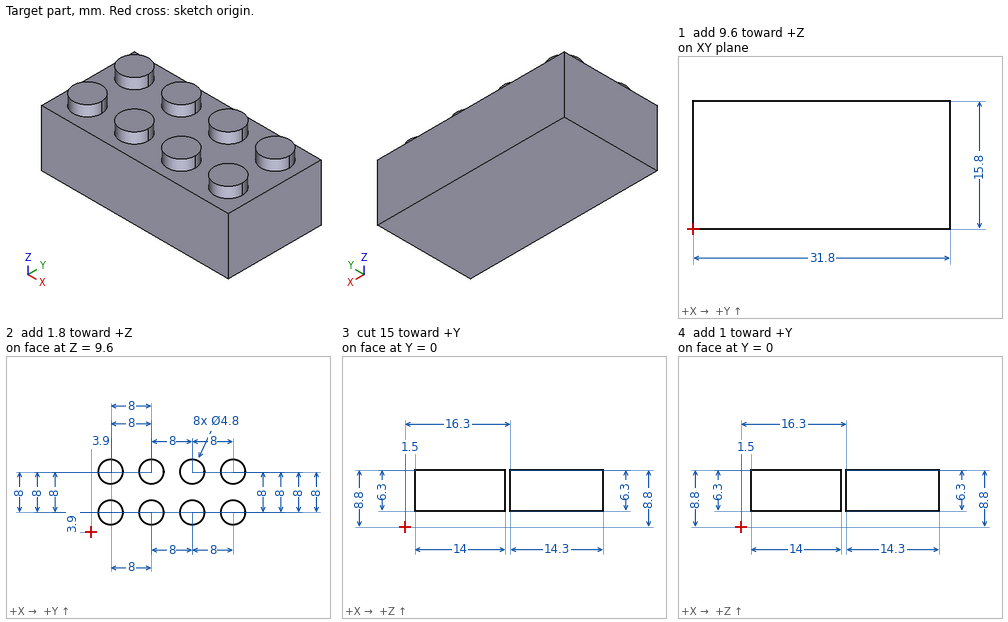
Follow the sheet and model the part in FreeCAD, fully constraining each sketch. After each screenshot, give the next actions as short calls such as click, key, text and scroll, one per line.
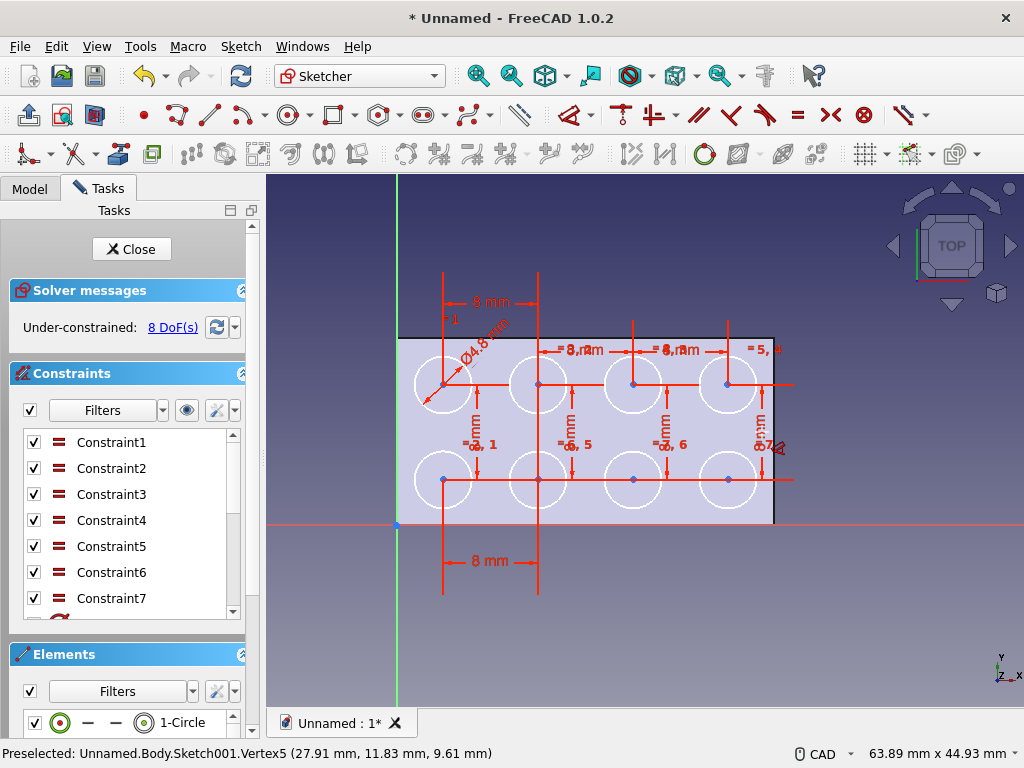
click(443, 480)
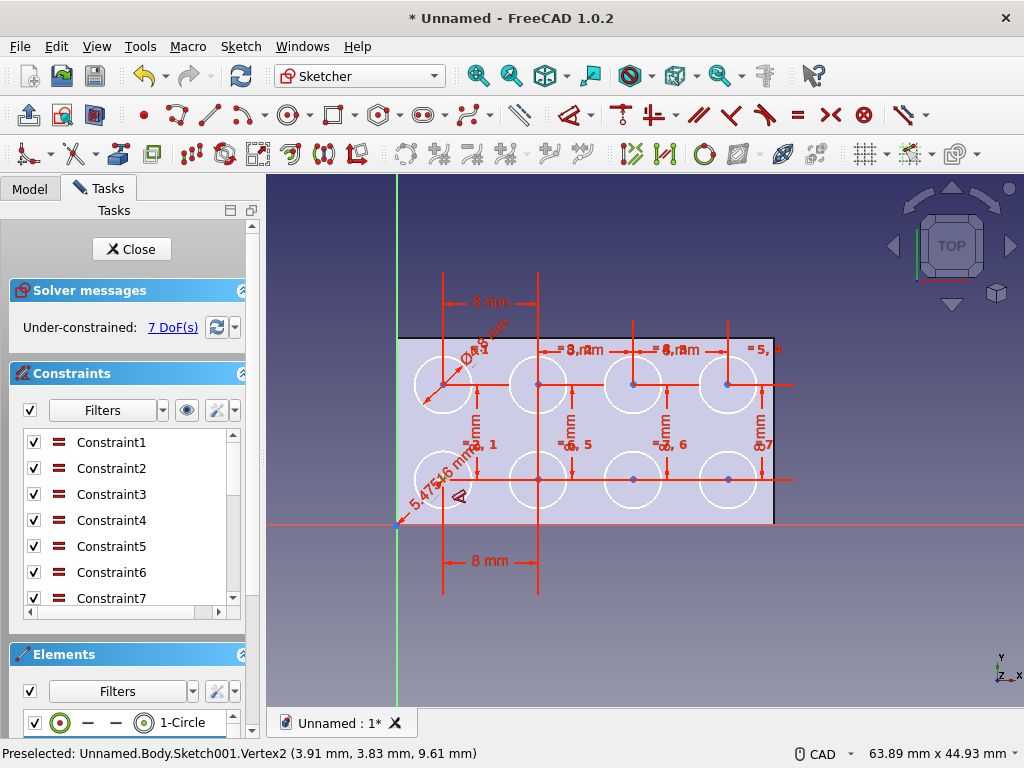
click(538, 480)
click(491, 398)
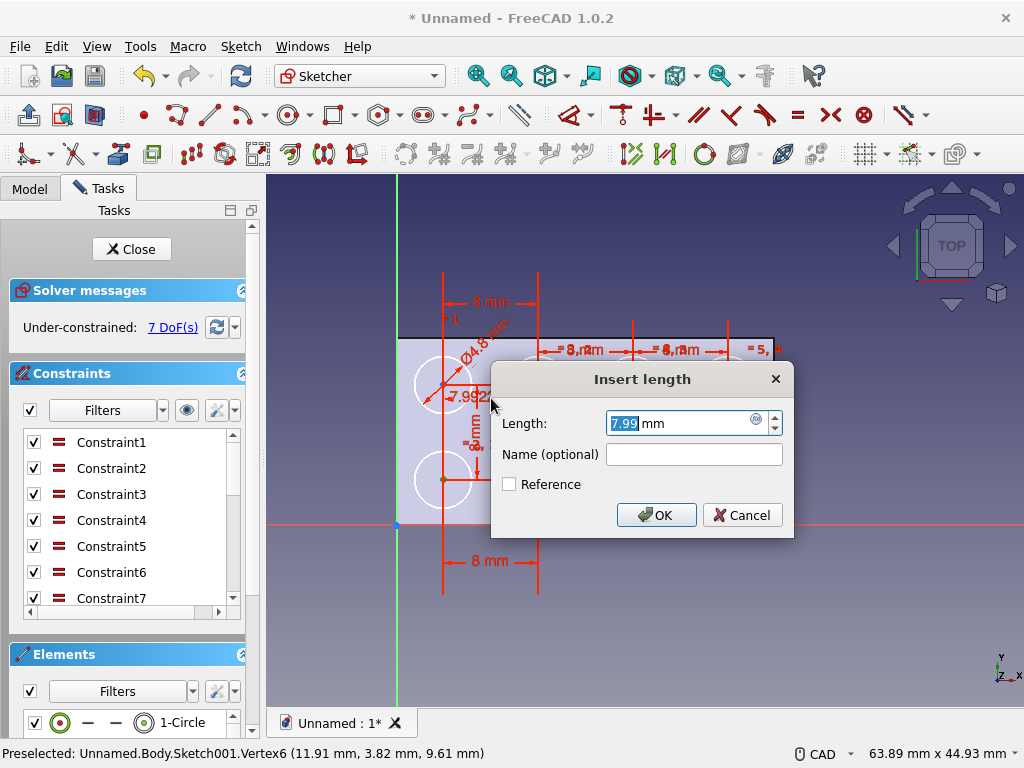
text(8)
key(Return)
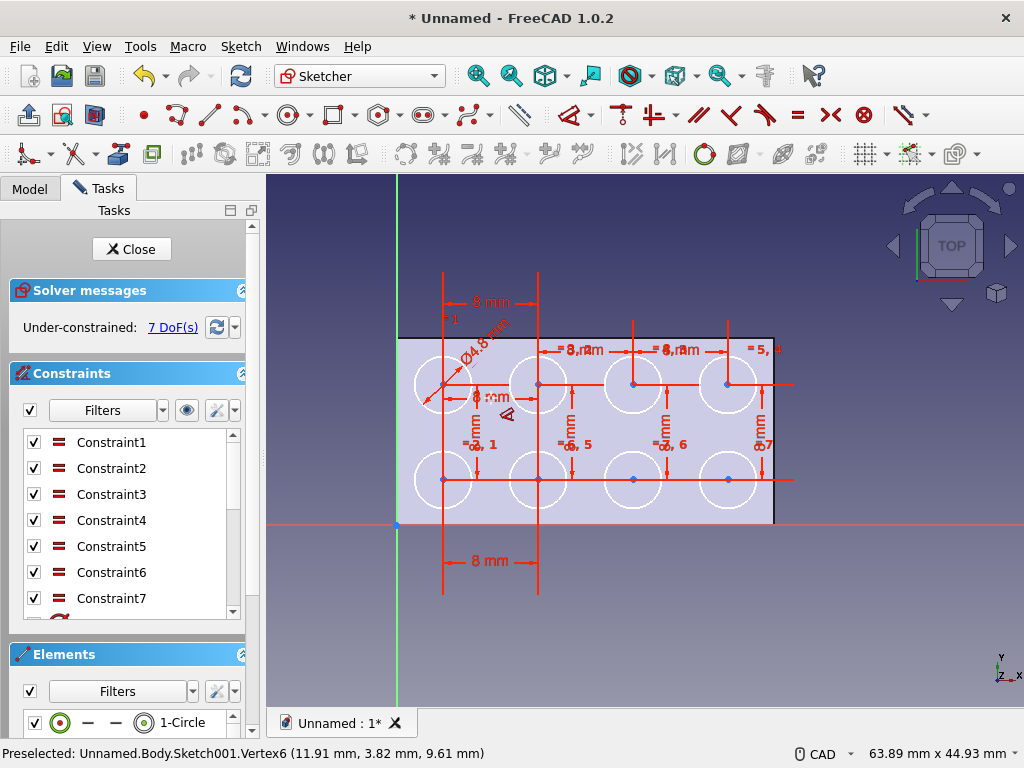
click(538, 385)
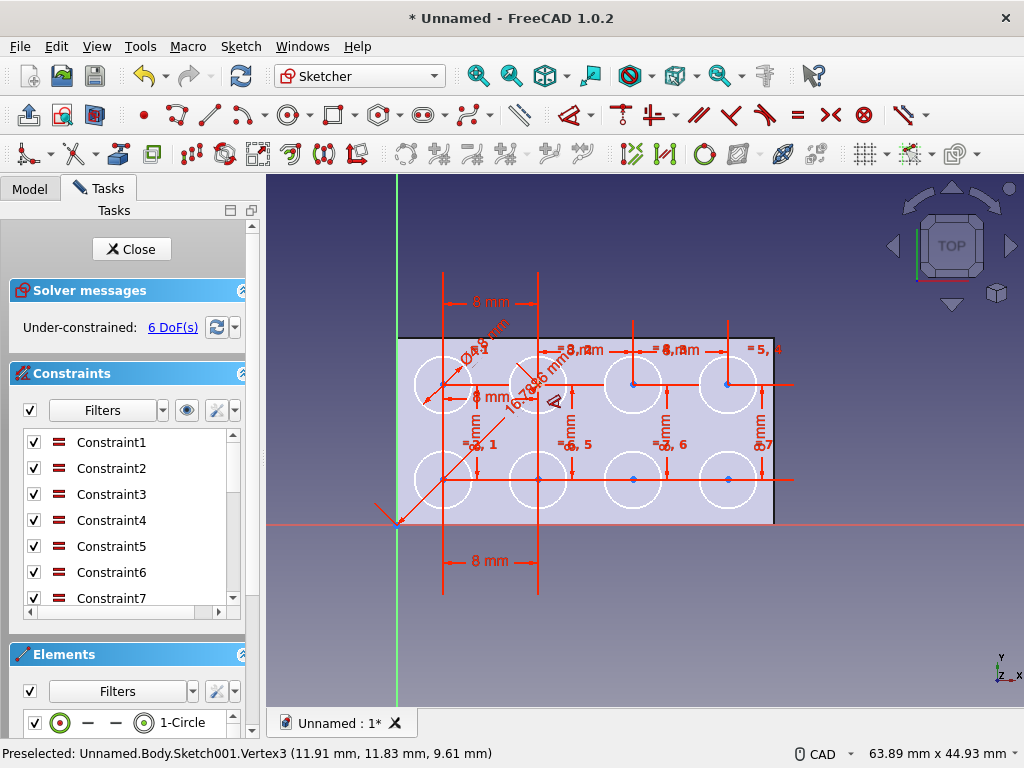
click(538, 480)
click(504, 454)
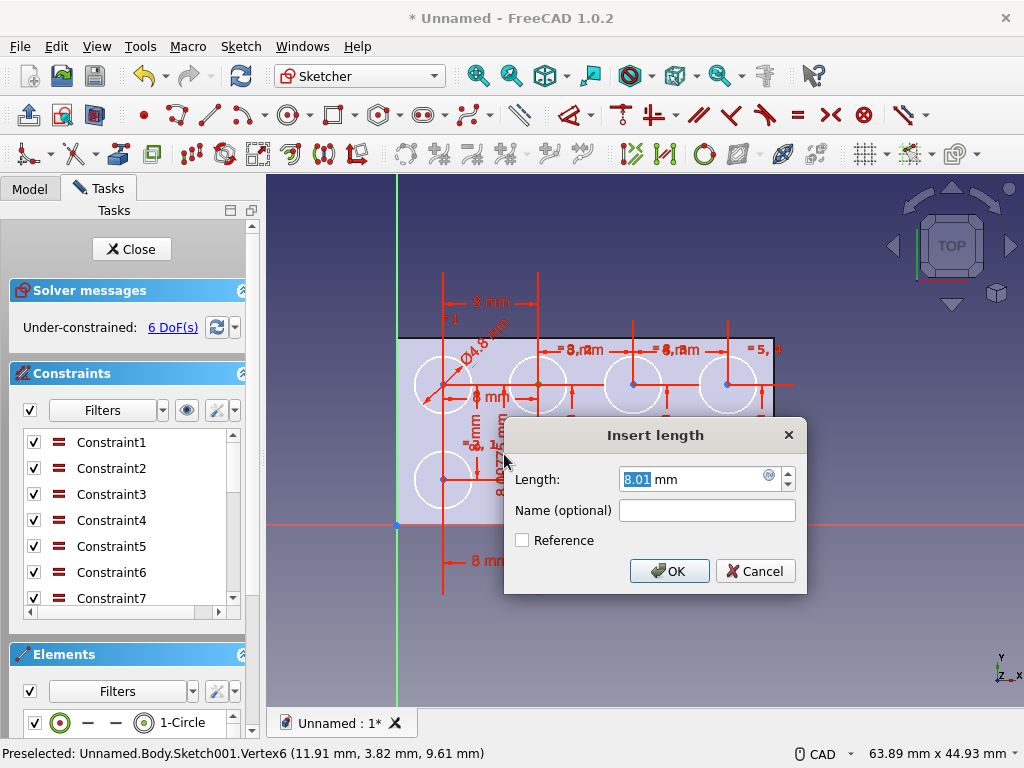
text(8)
key(Return)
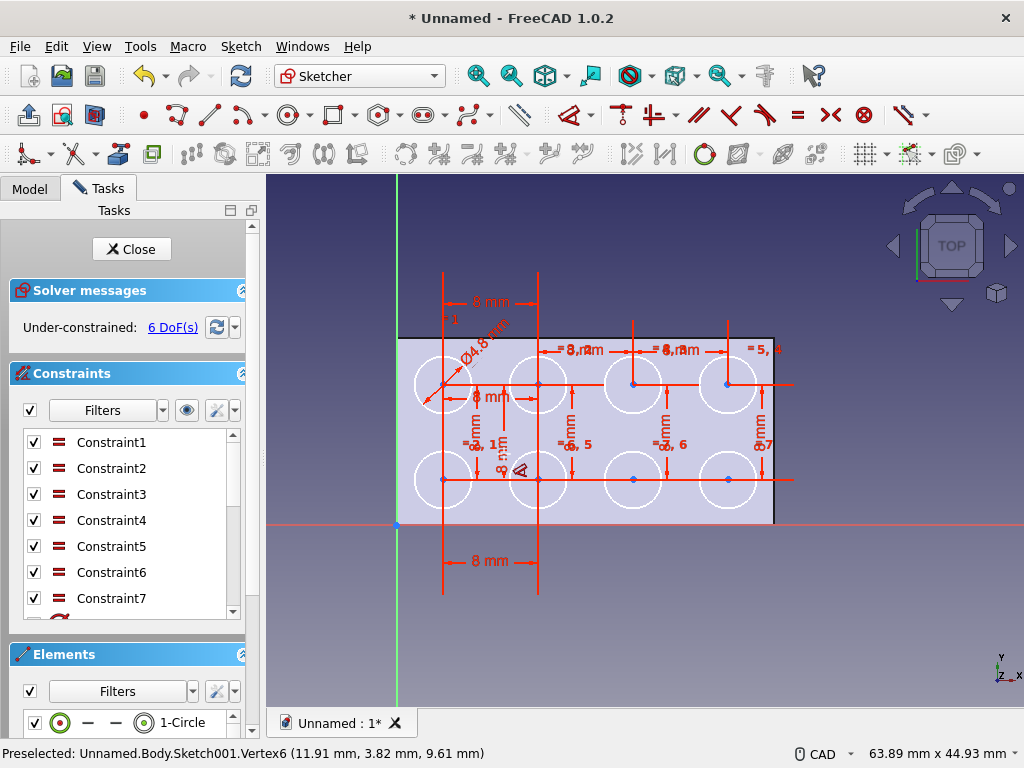
click(538, 480)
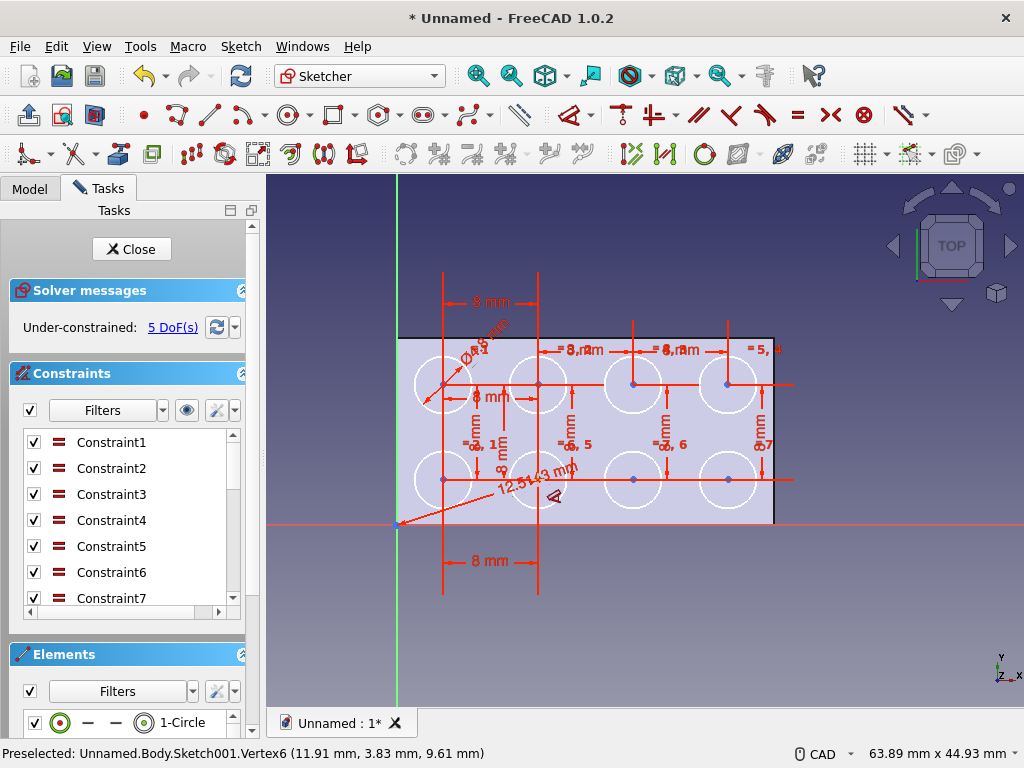
click(633, 480)
click(586, 562)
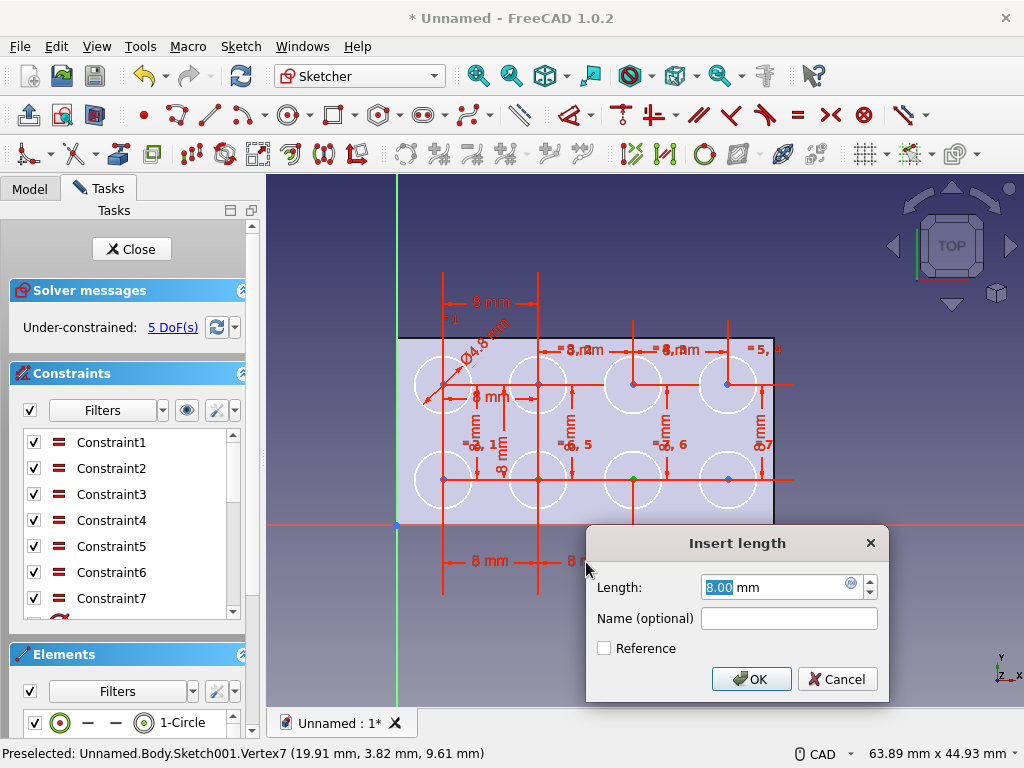
text(8)
key(Return)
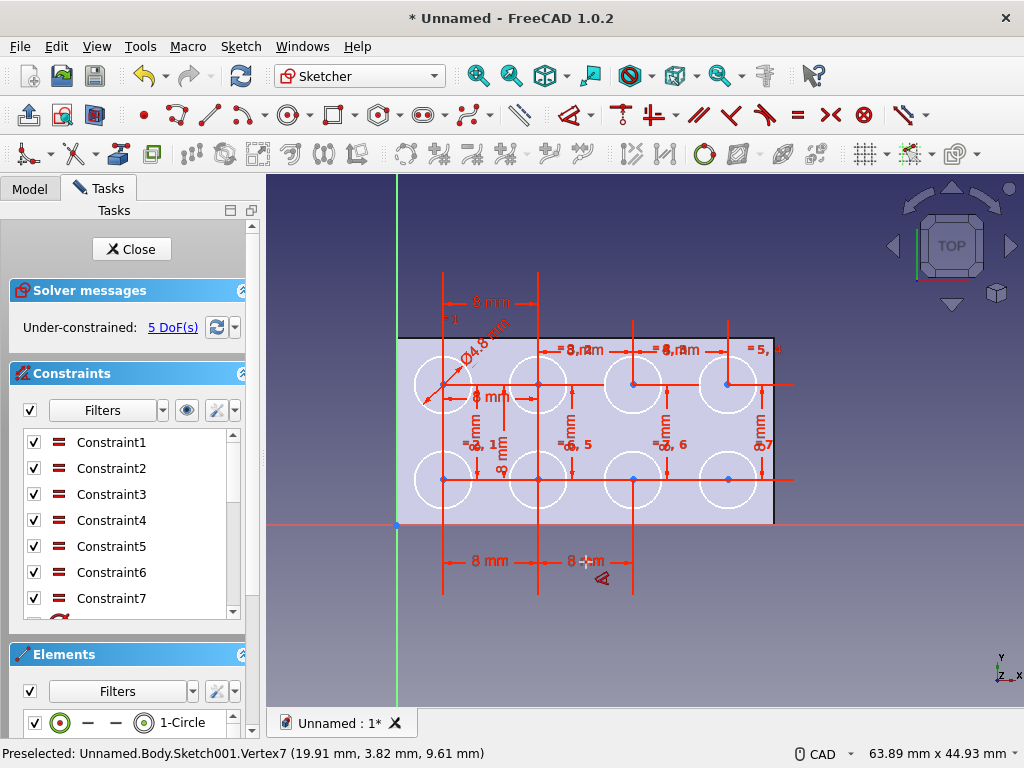
click(633, 385)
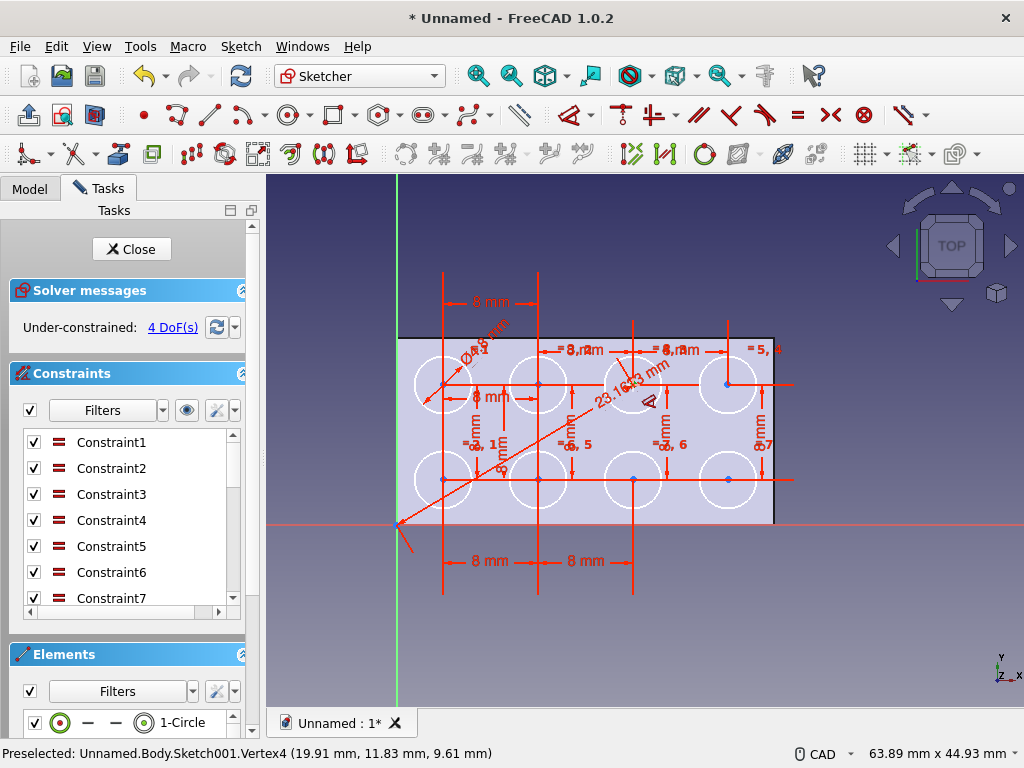
click(633, 480)
click(667, 411)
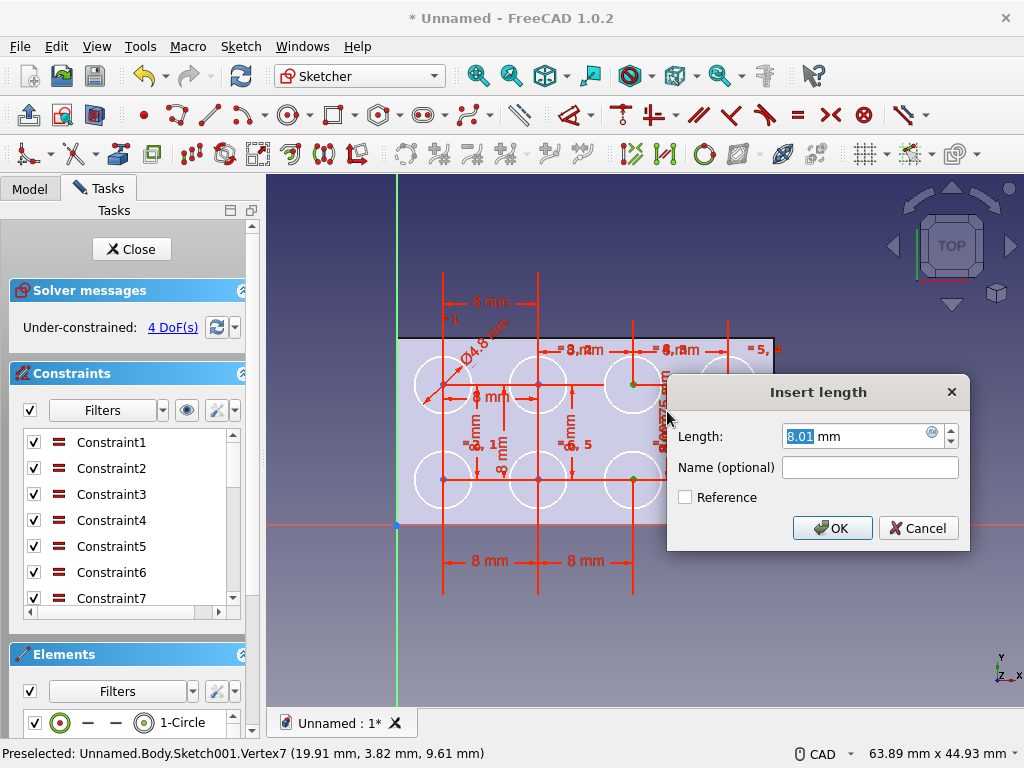
text(8)
key(Return)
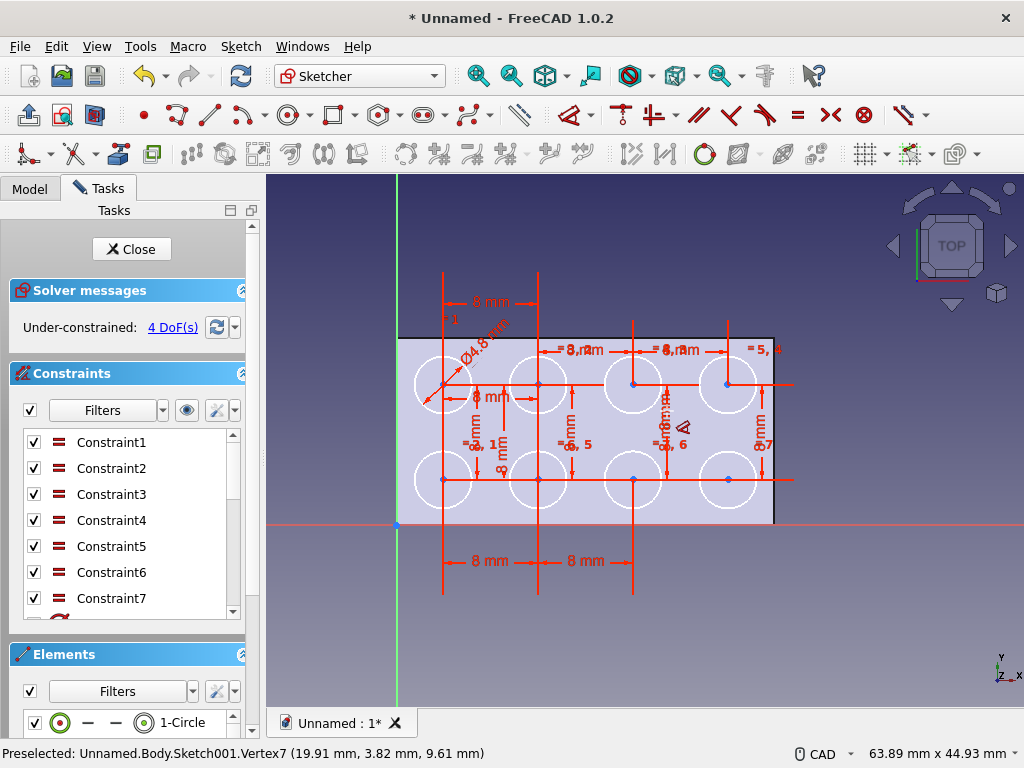
click(633, 480)